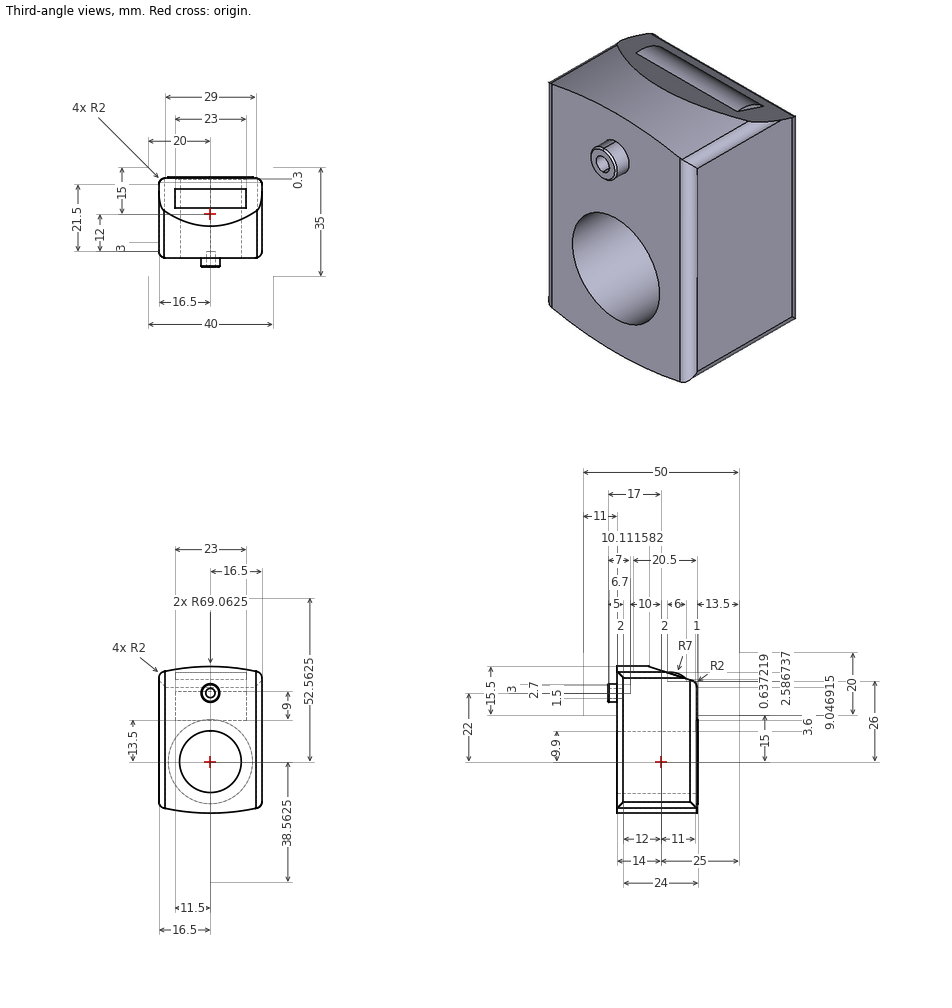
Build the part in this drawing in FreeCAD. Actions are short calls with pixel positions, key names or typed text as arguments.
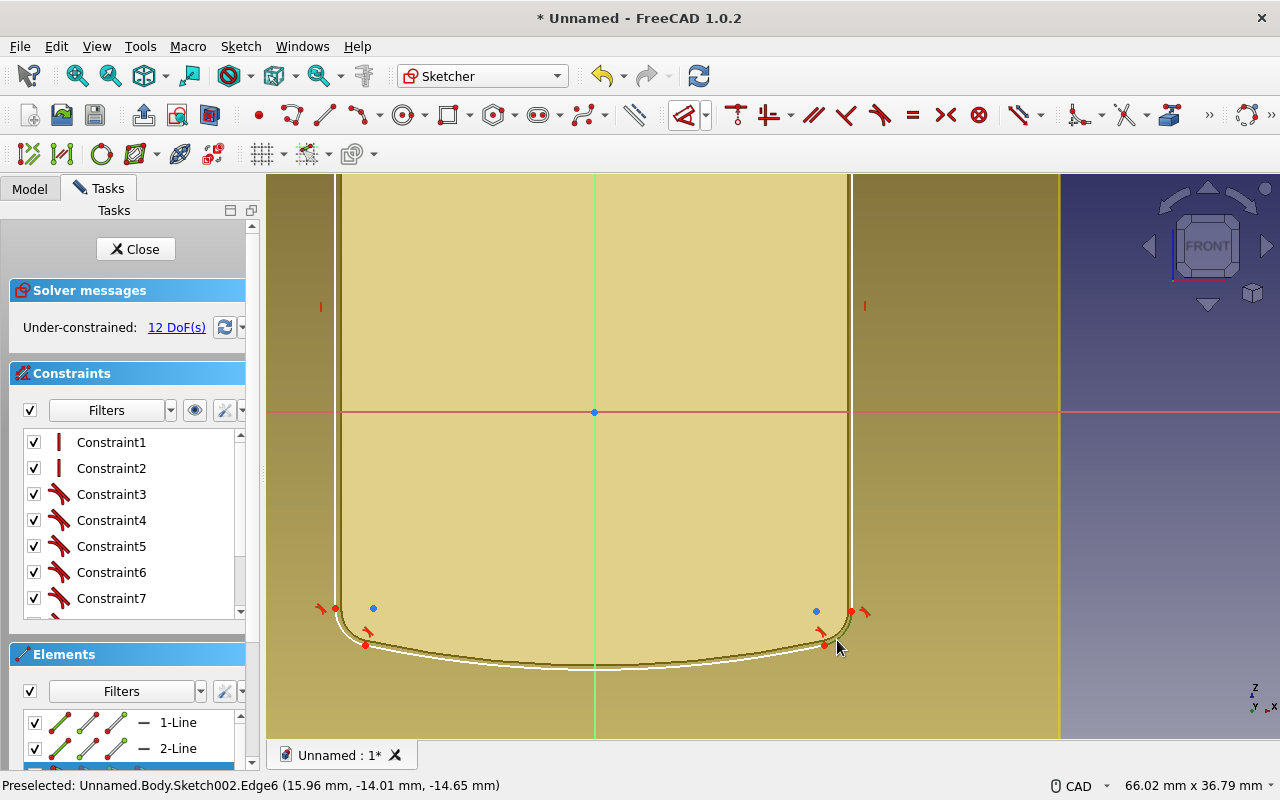
click(338, 623)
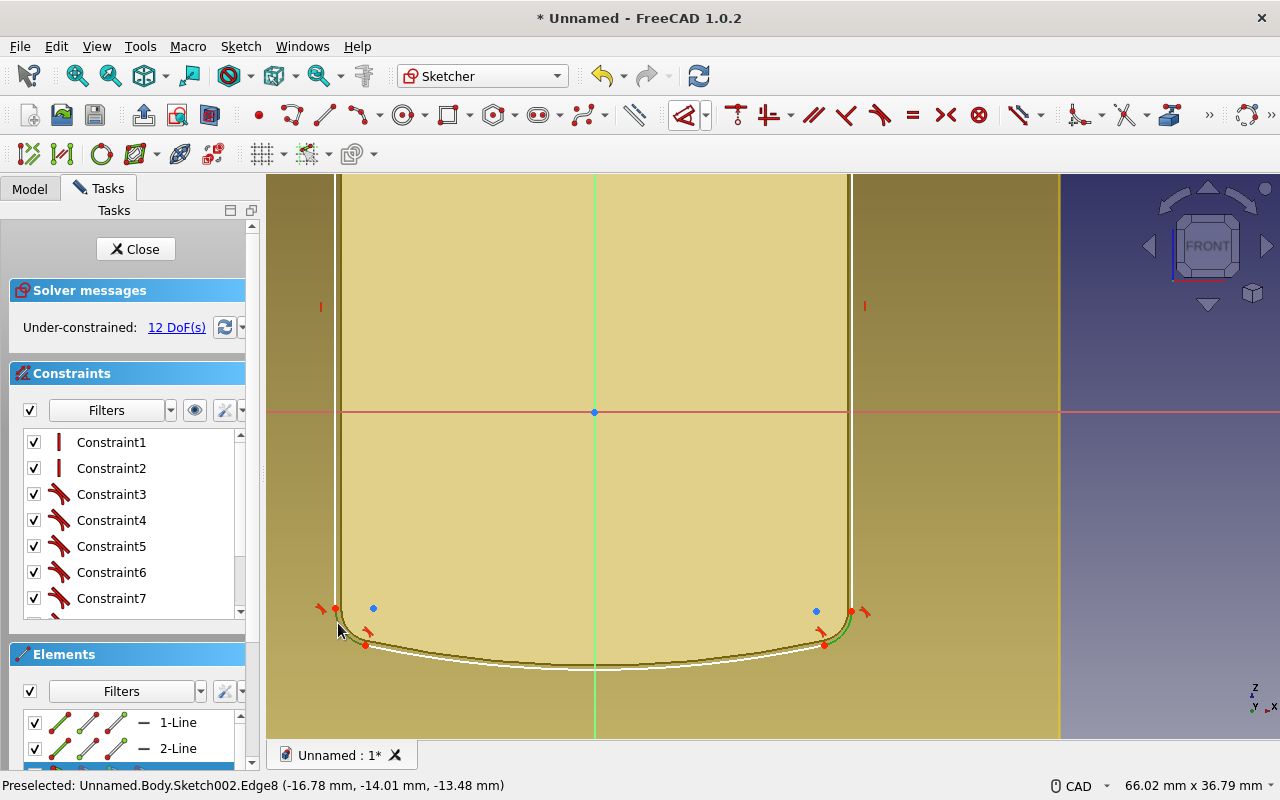
click(913, 116)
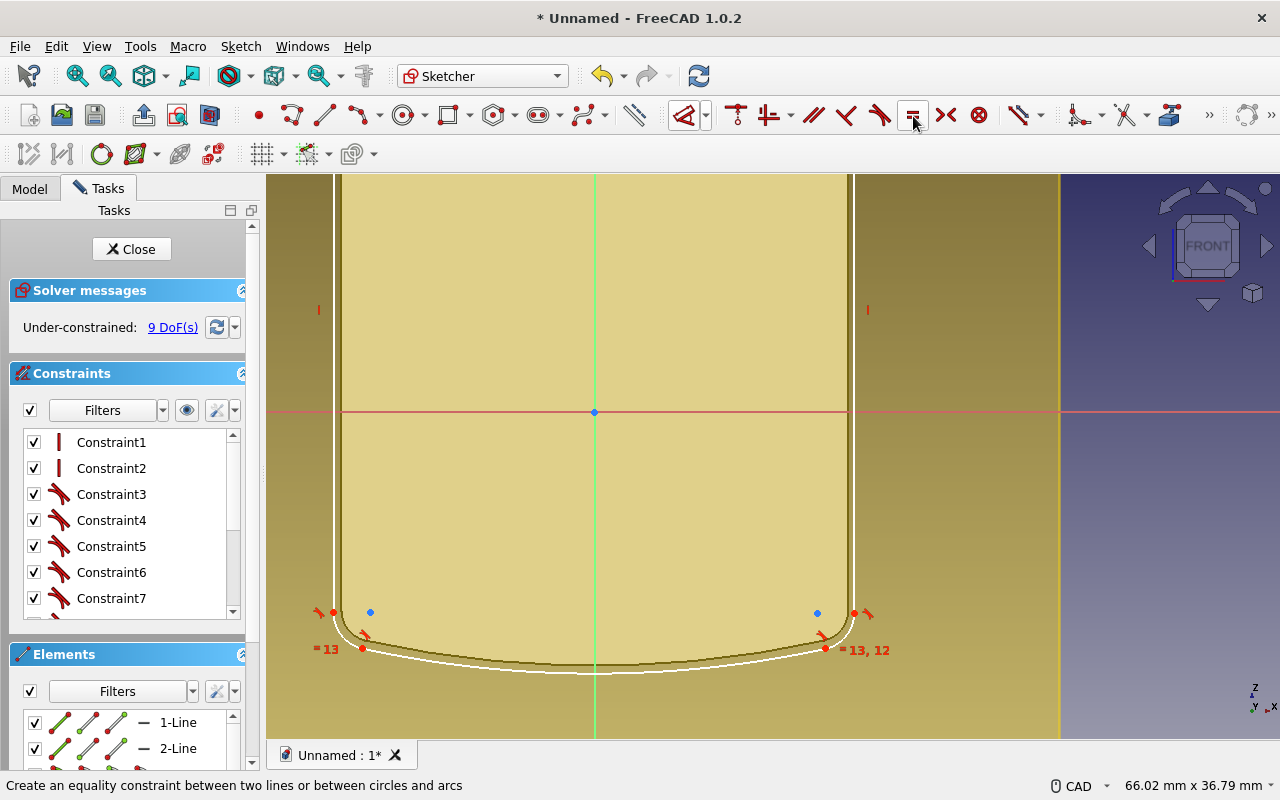
scroll(838, 641, down, 3)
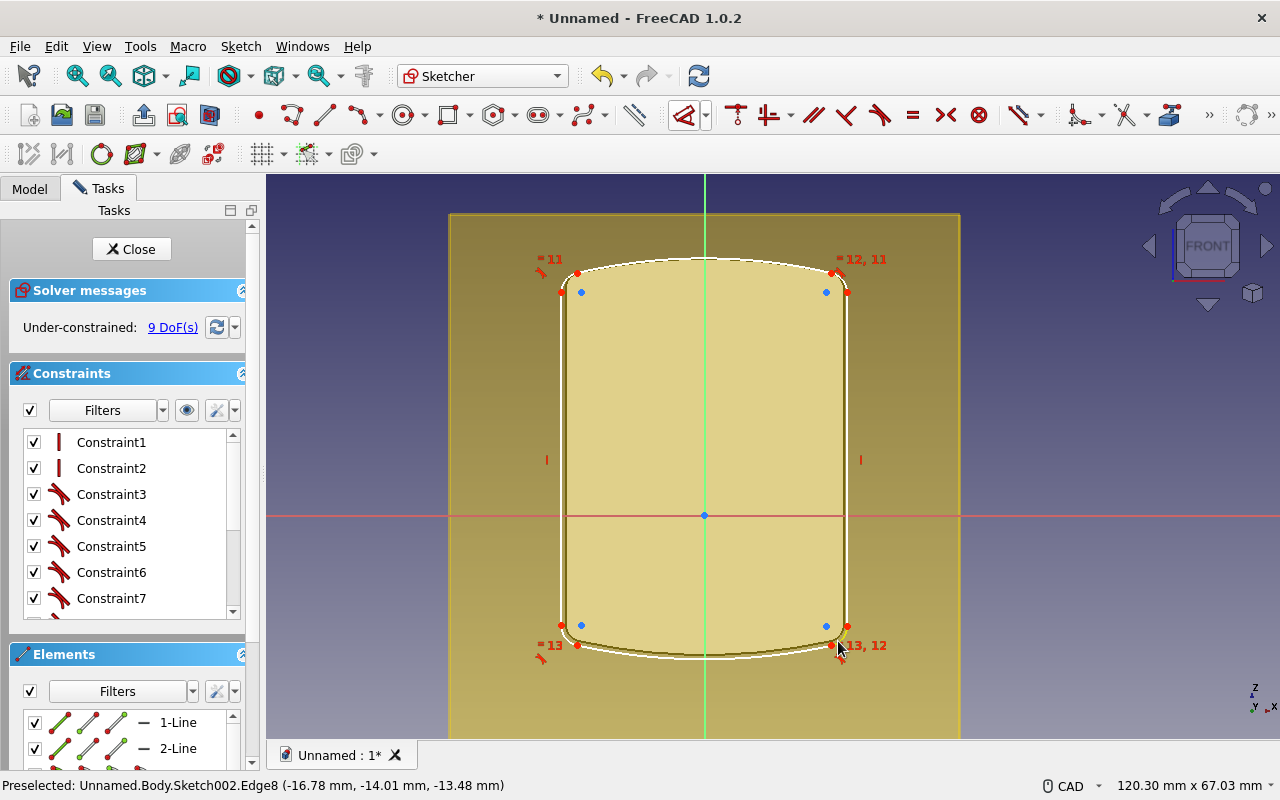
click(756, 261)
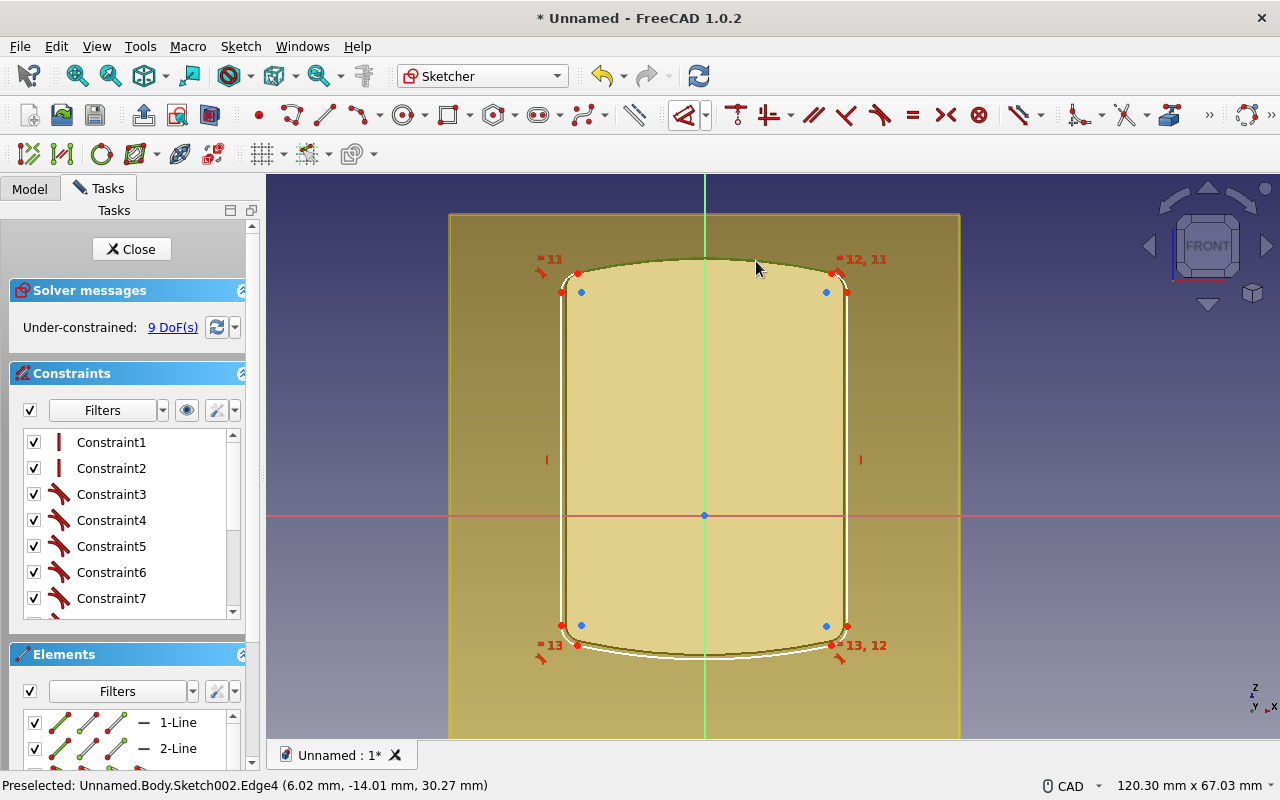
click(653, 657)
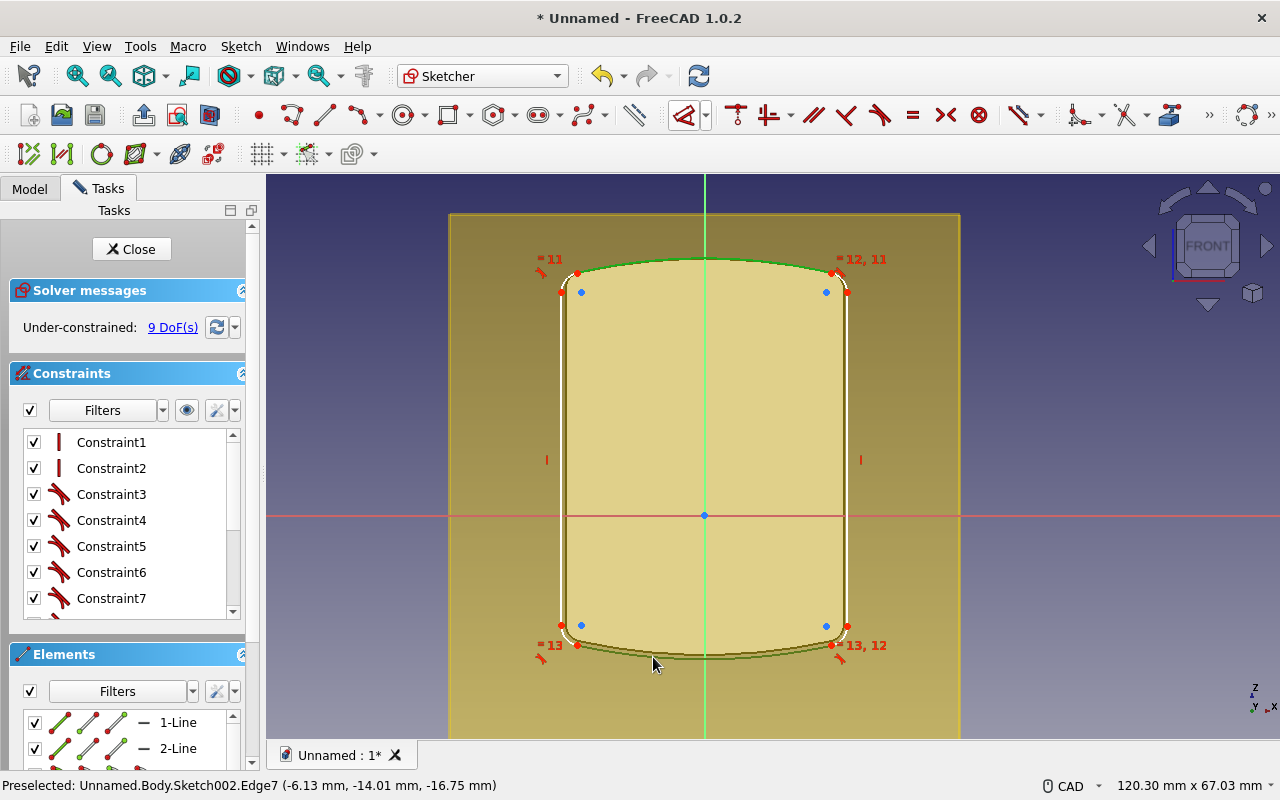
click(913, 116)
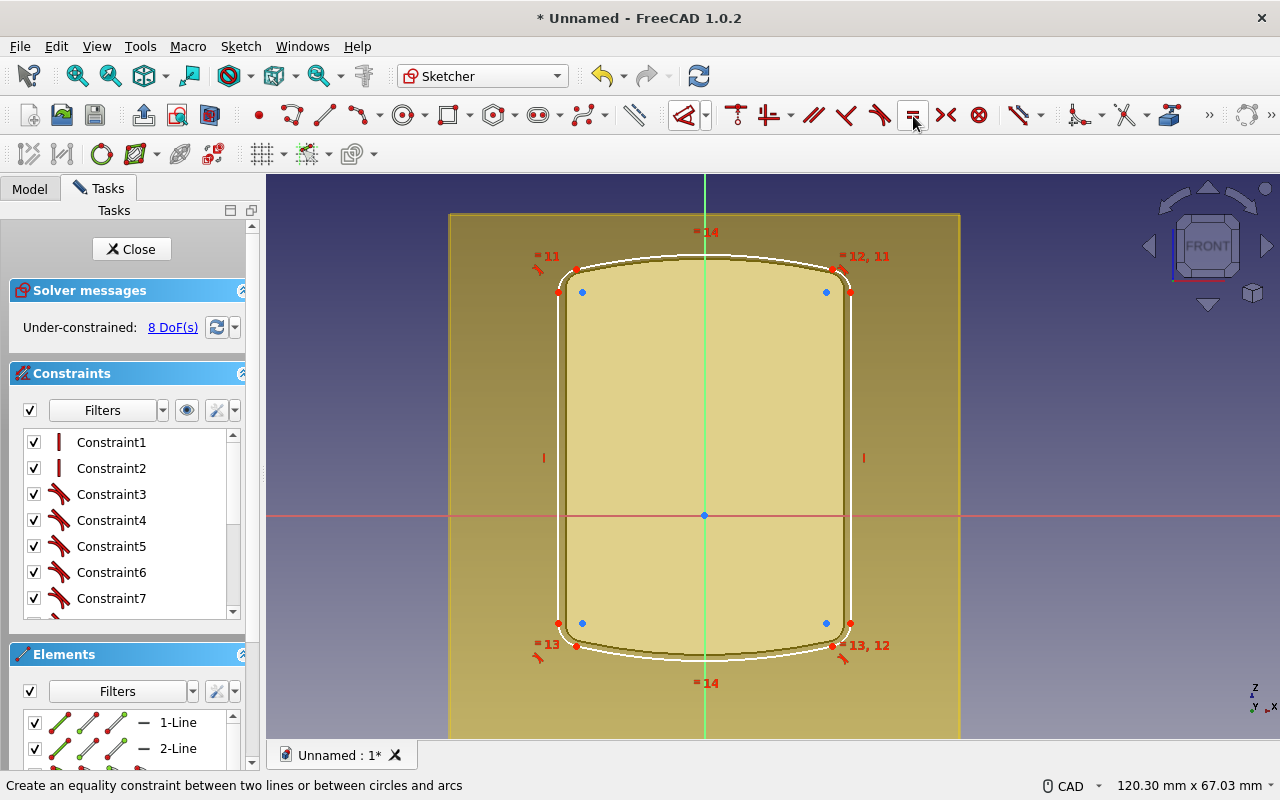
scroll(704, 291, down, 2)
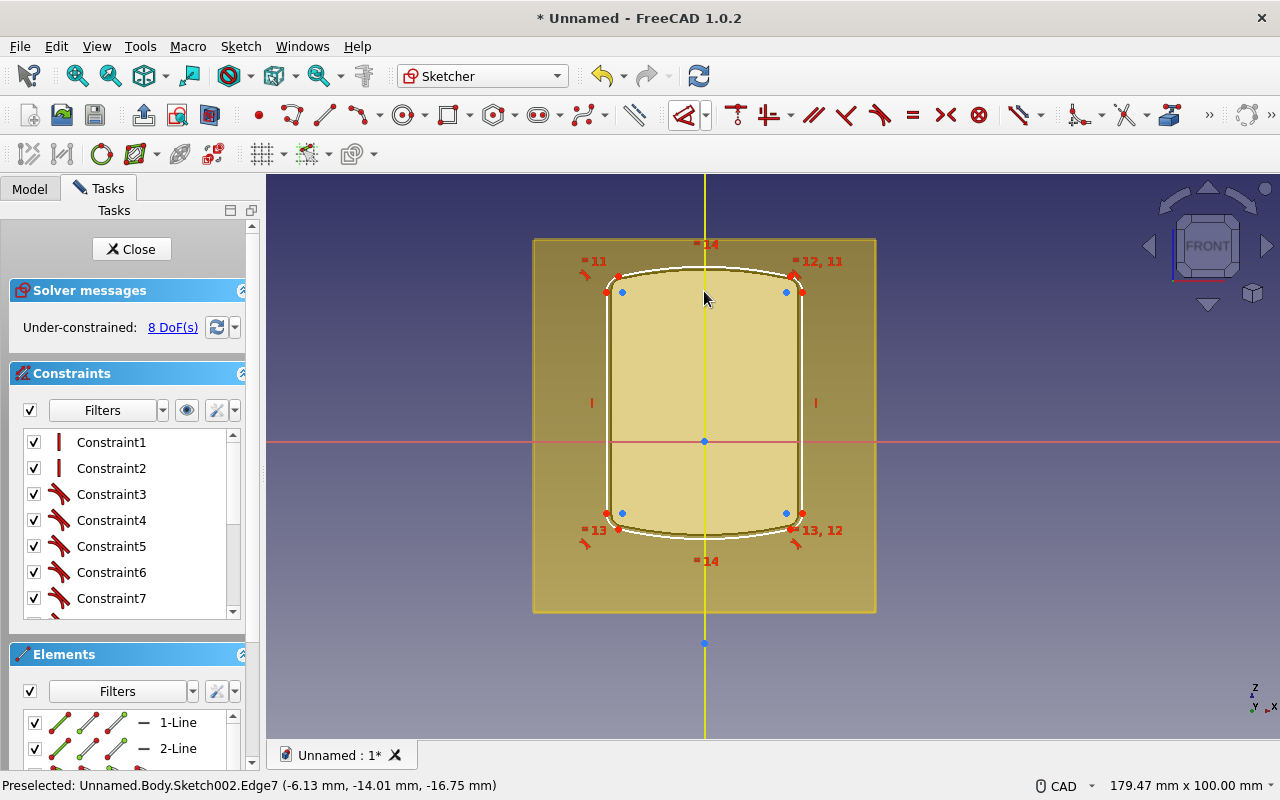
click(704, 644)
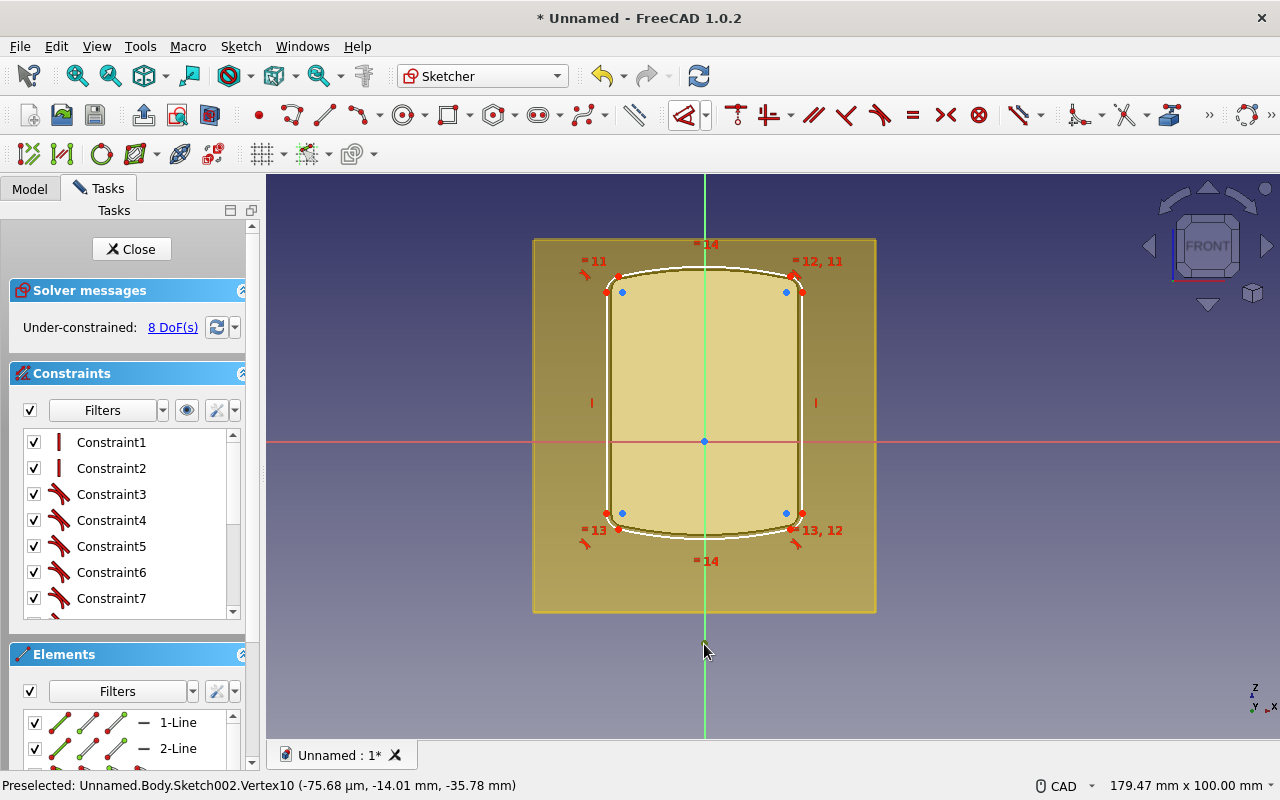
click(705, 675)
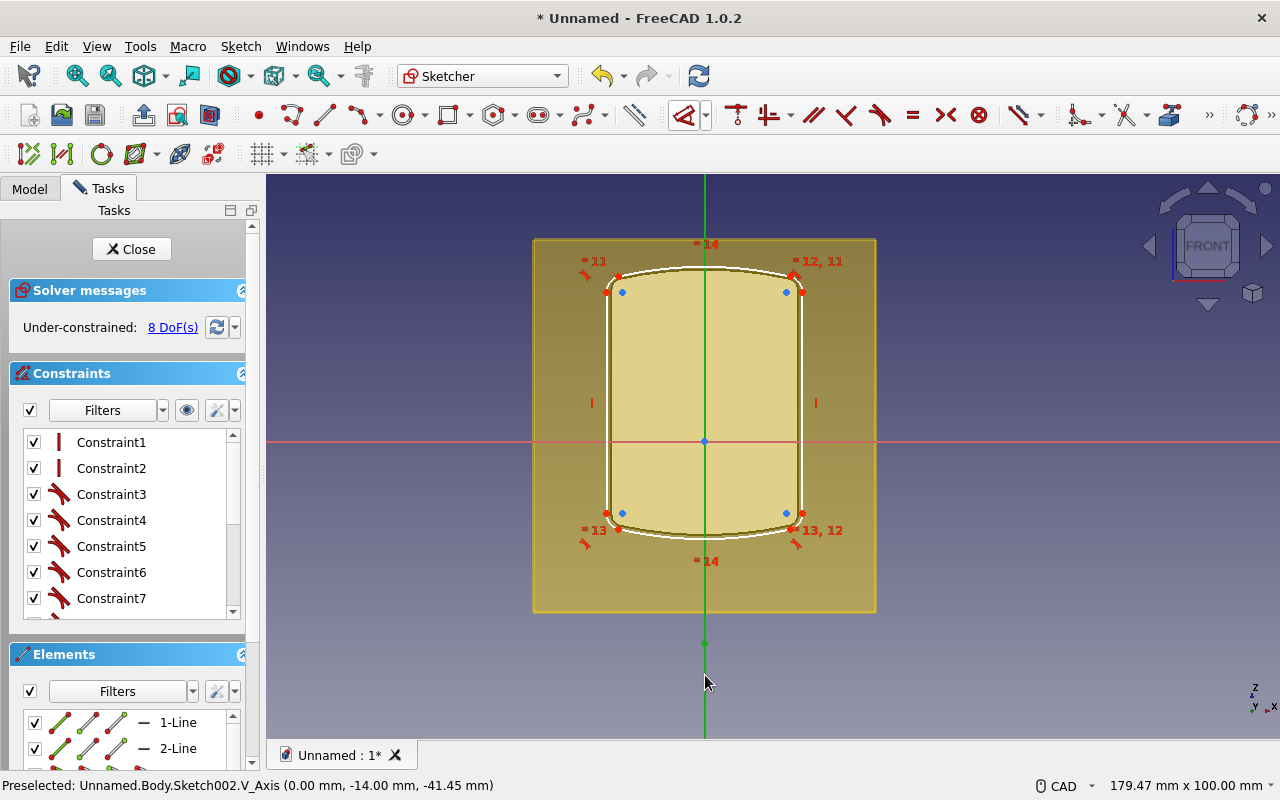
click(736, 116)